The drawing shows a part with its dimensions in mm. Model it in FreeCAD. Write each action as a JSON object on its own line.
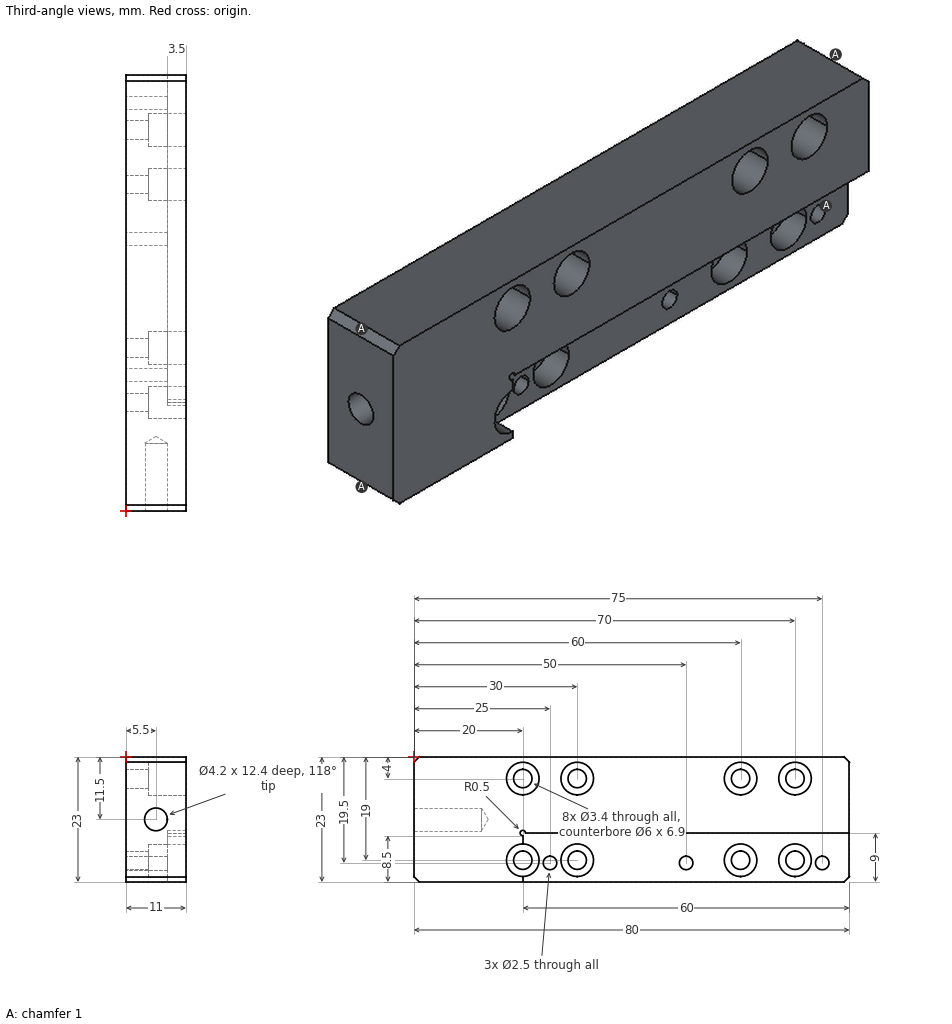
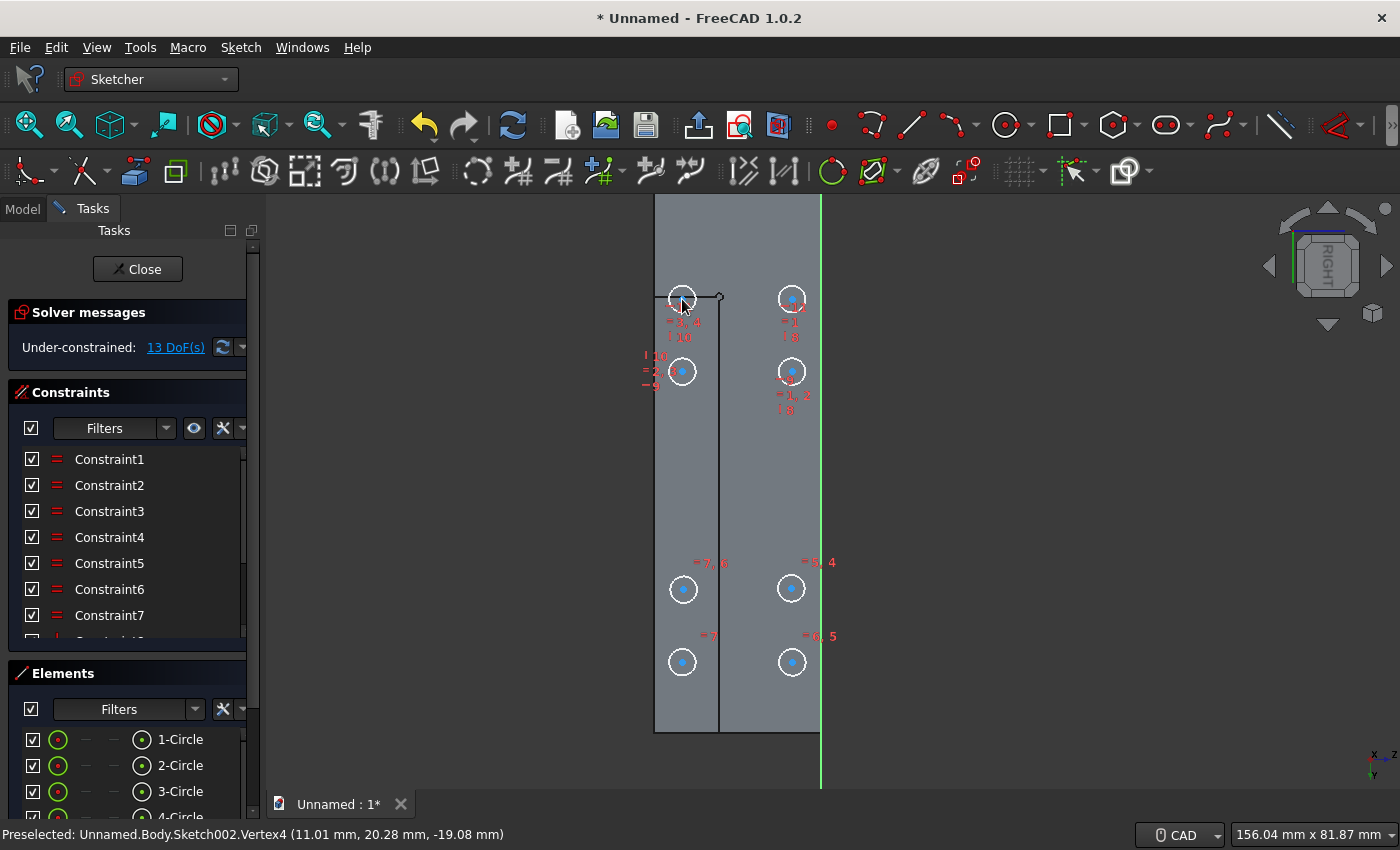
{"action": "left_click", "coordinate": [792, 372]}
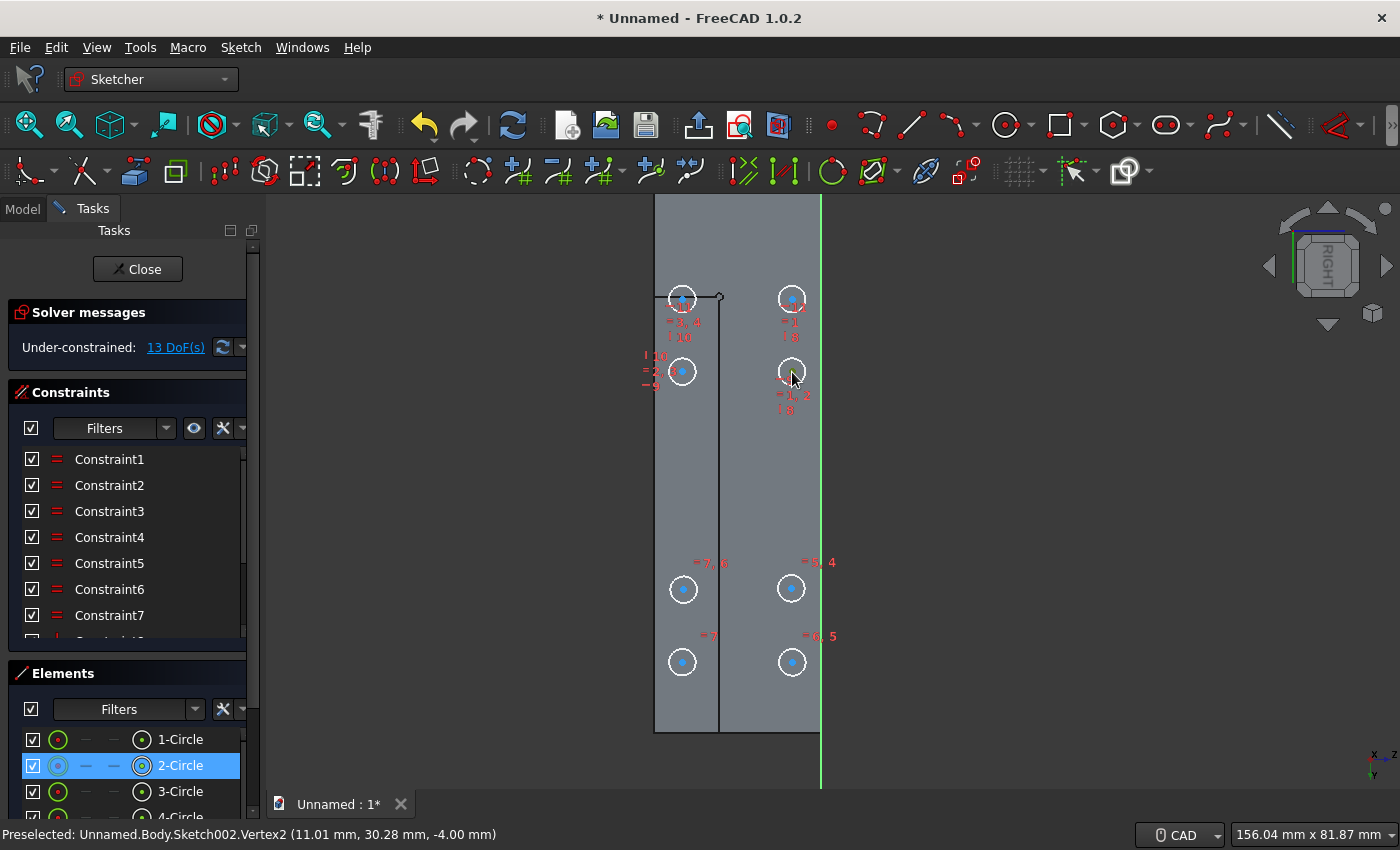
{"action": "left_click", "coordinate": [791, 588]}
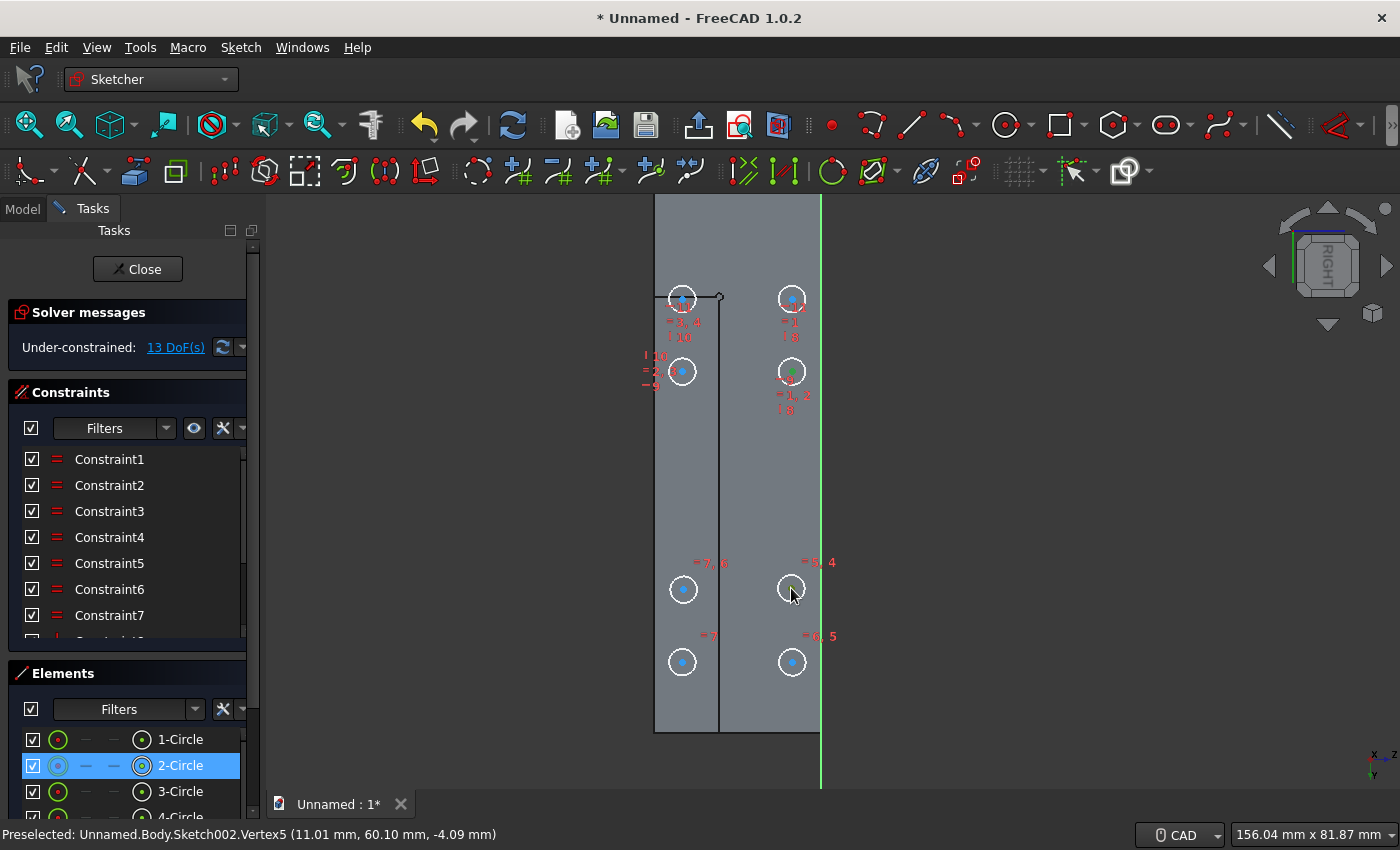
{"action": "key", "text": "v"}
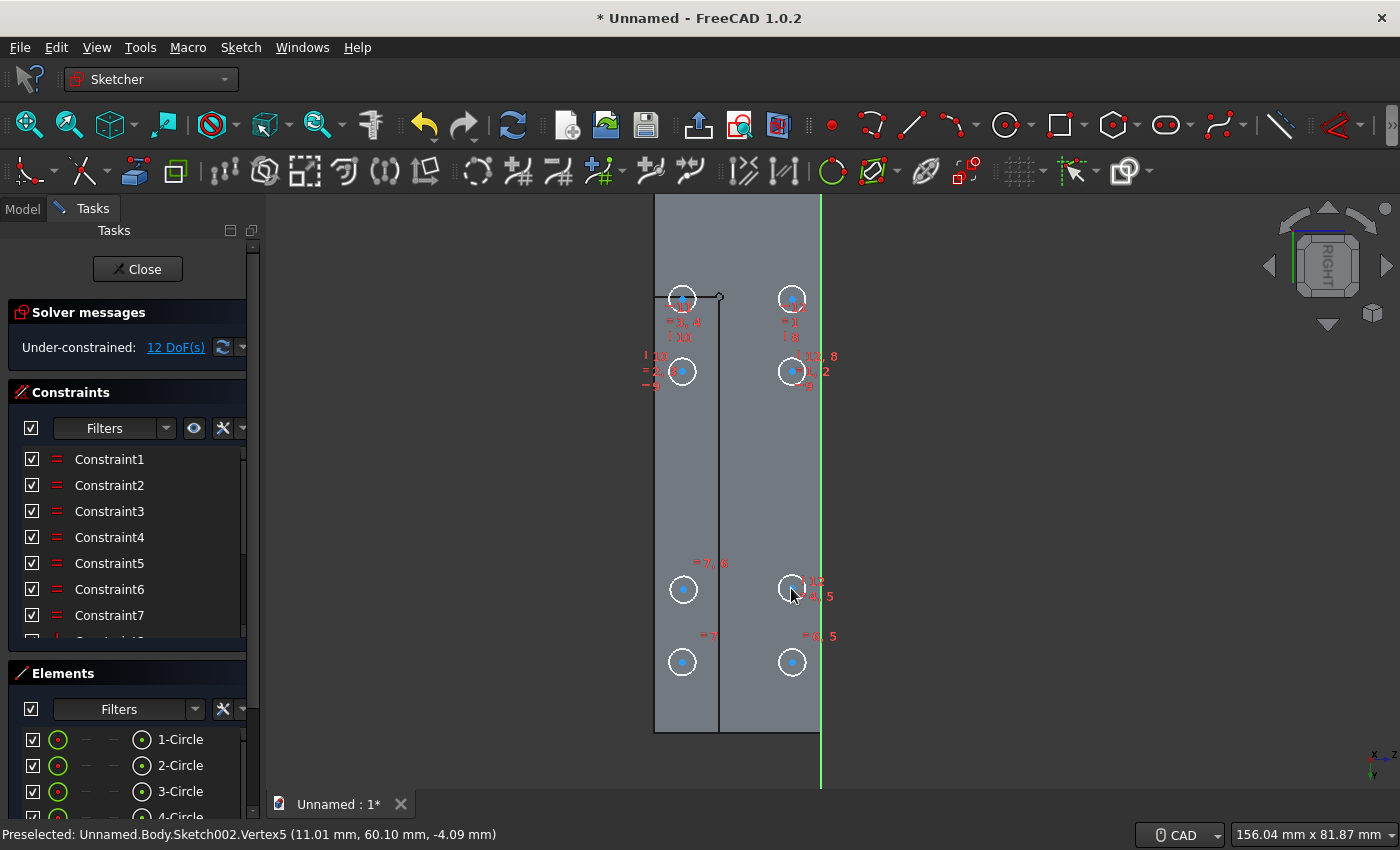
{"action": "left_click", "coordinate": [792, 588]}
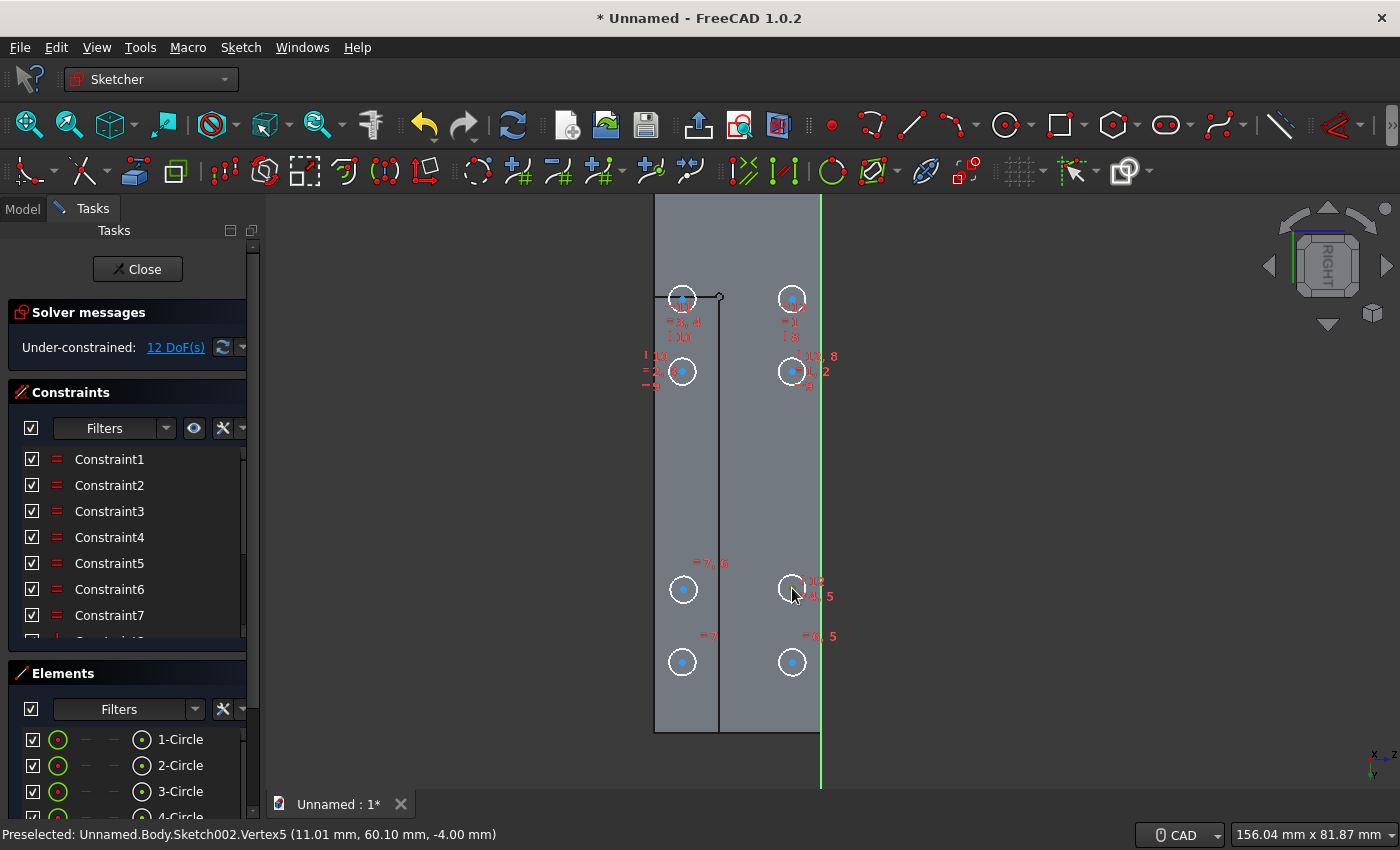
{"action": "left_click", "coordinate": [792, 662]}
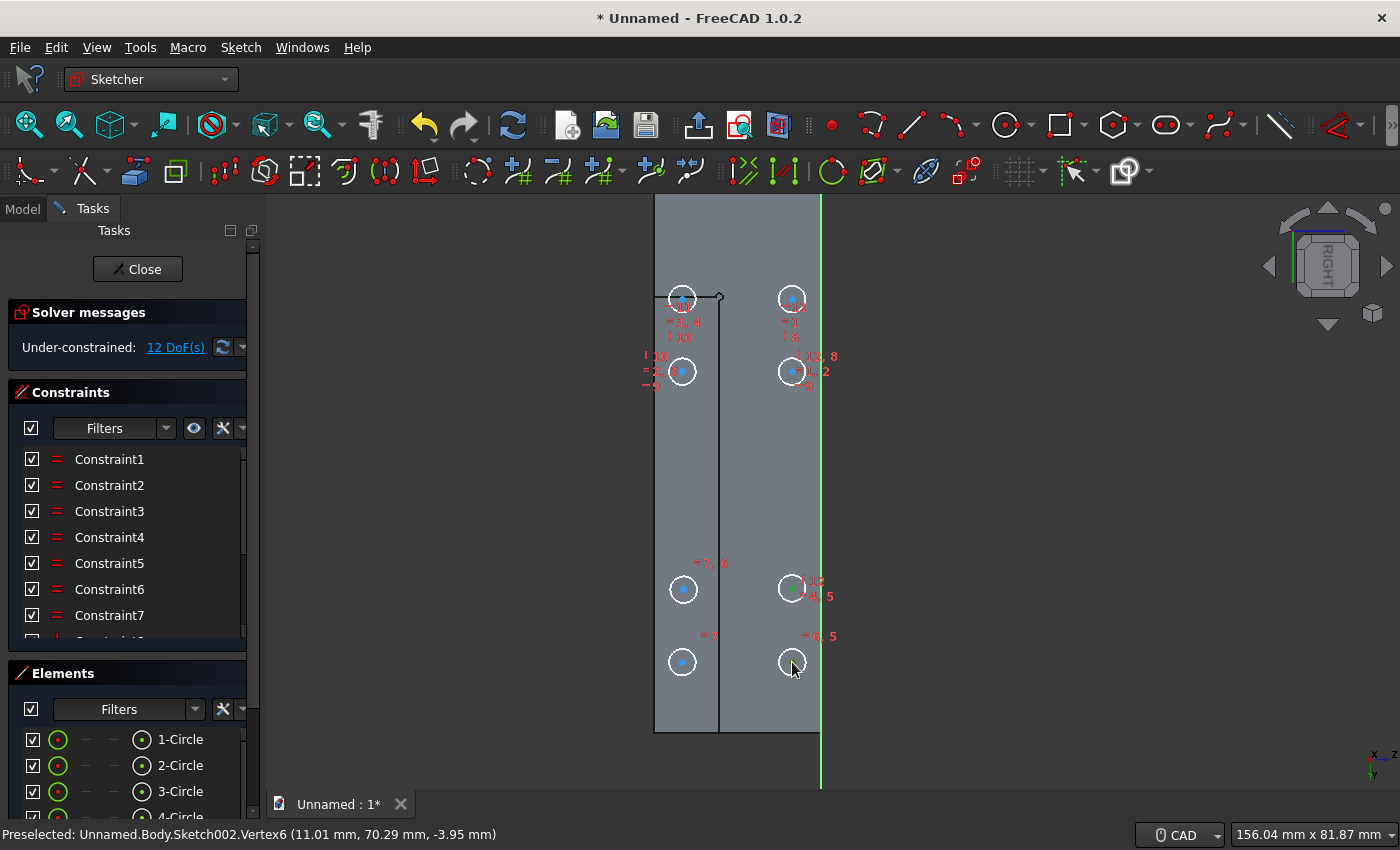
{"action": "key", "text": "v"}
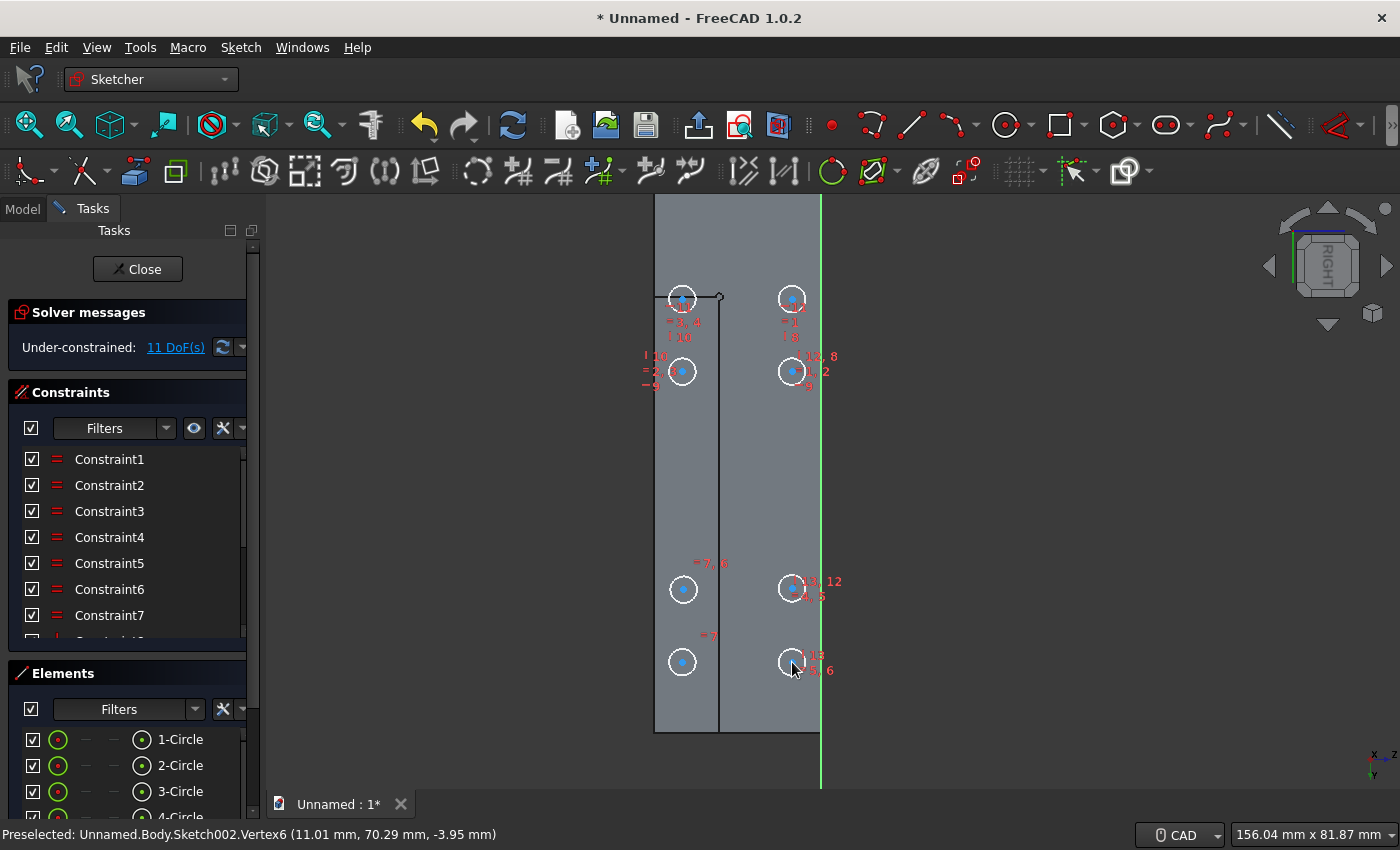
{"action": "left_click", "coordinate": [682, 372]}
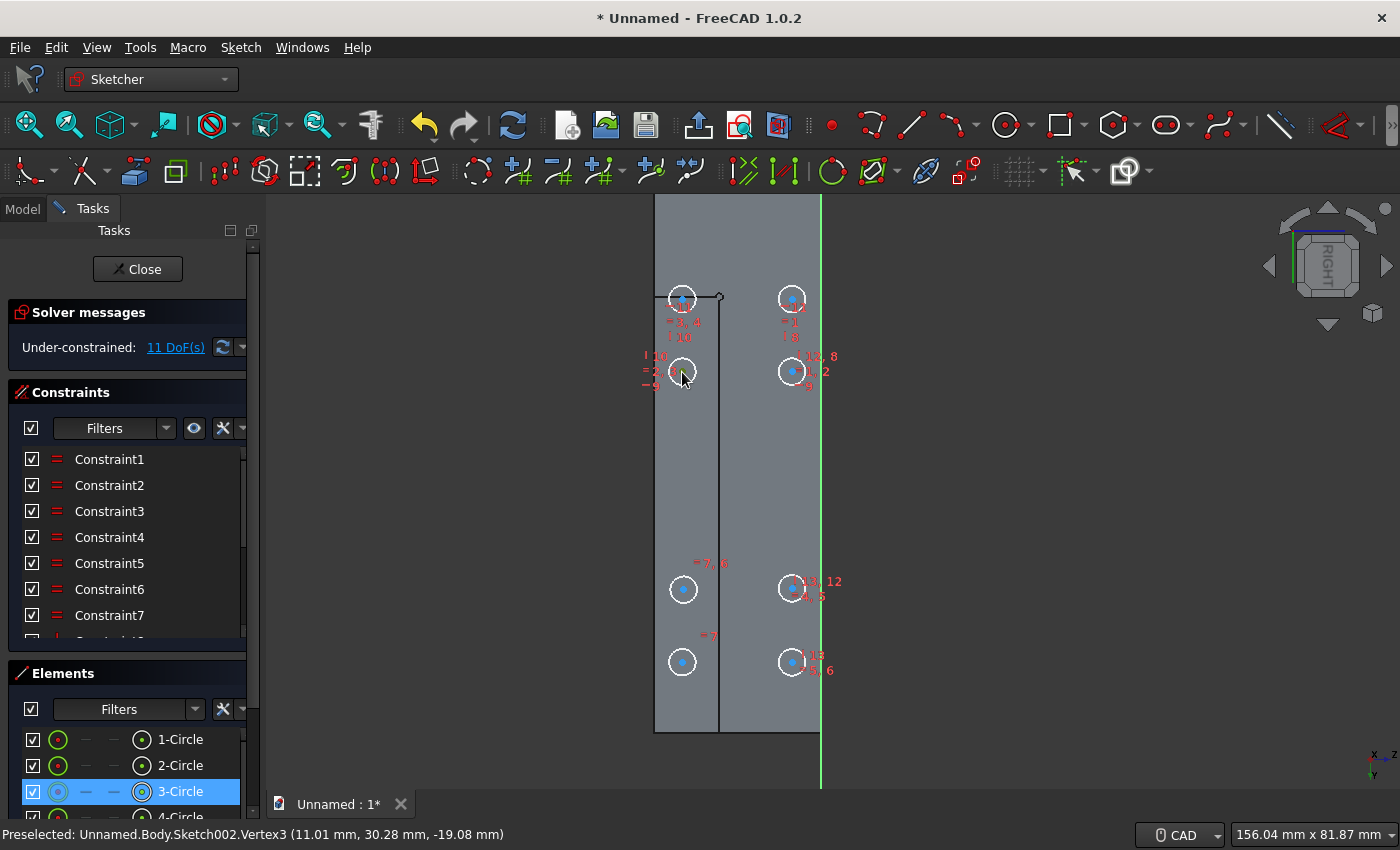
{"action": "left_click", "coordinate": [684, 590]}